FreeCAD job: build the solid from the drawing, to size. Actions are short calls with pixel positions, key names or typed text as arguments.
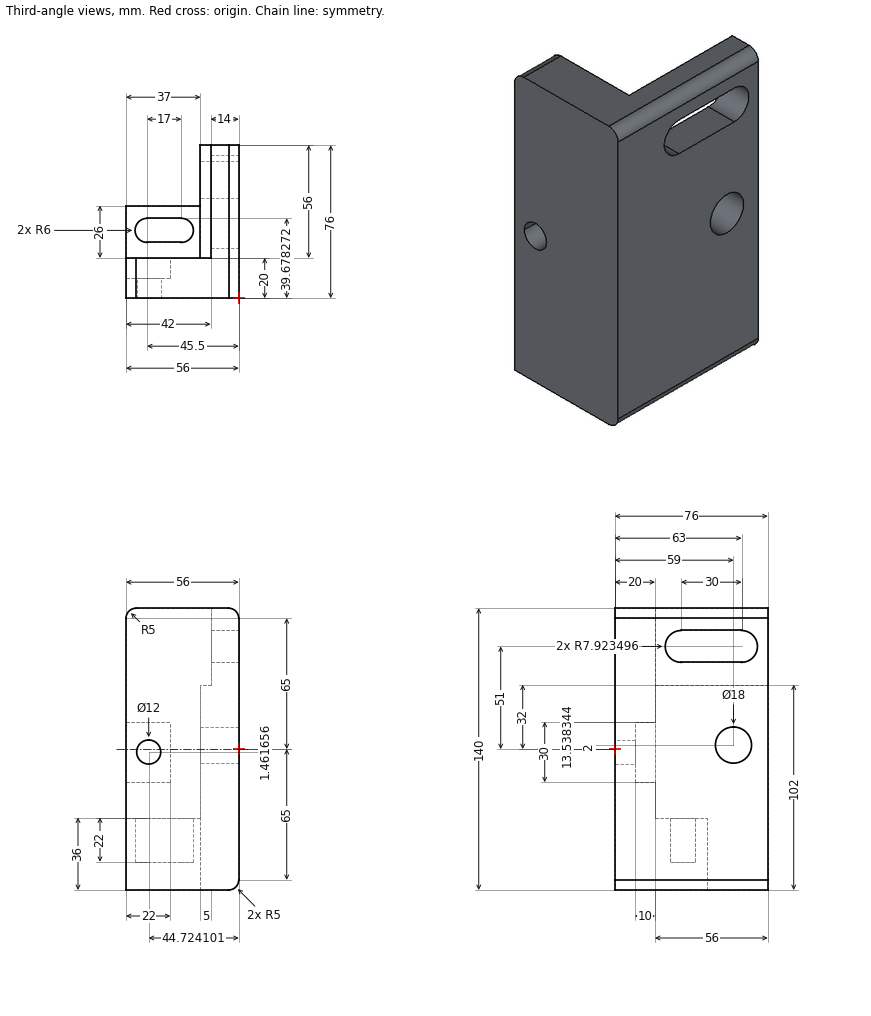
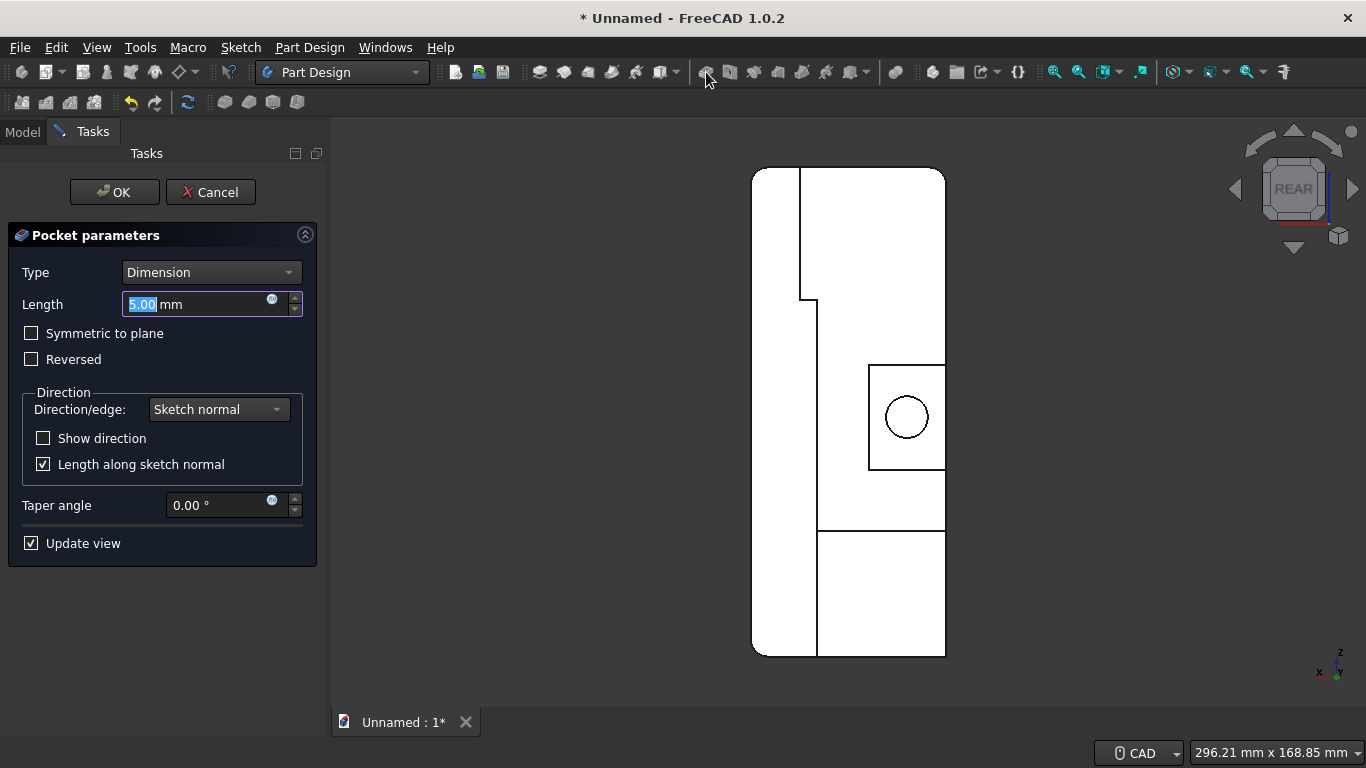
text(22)
key(Tab)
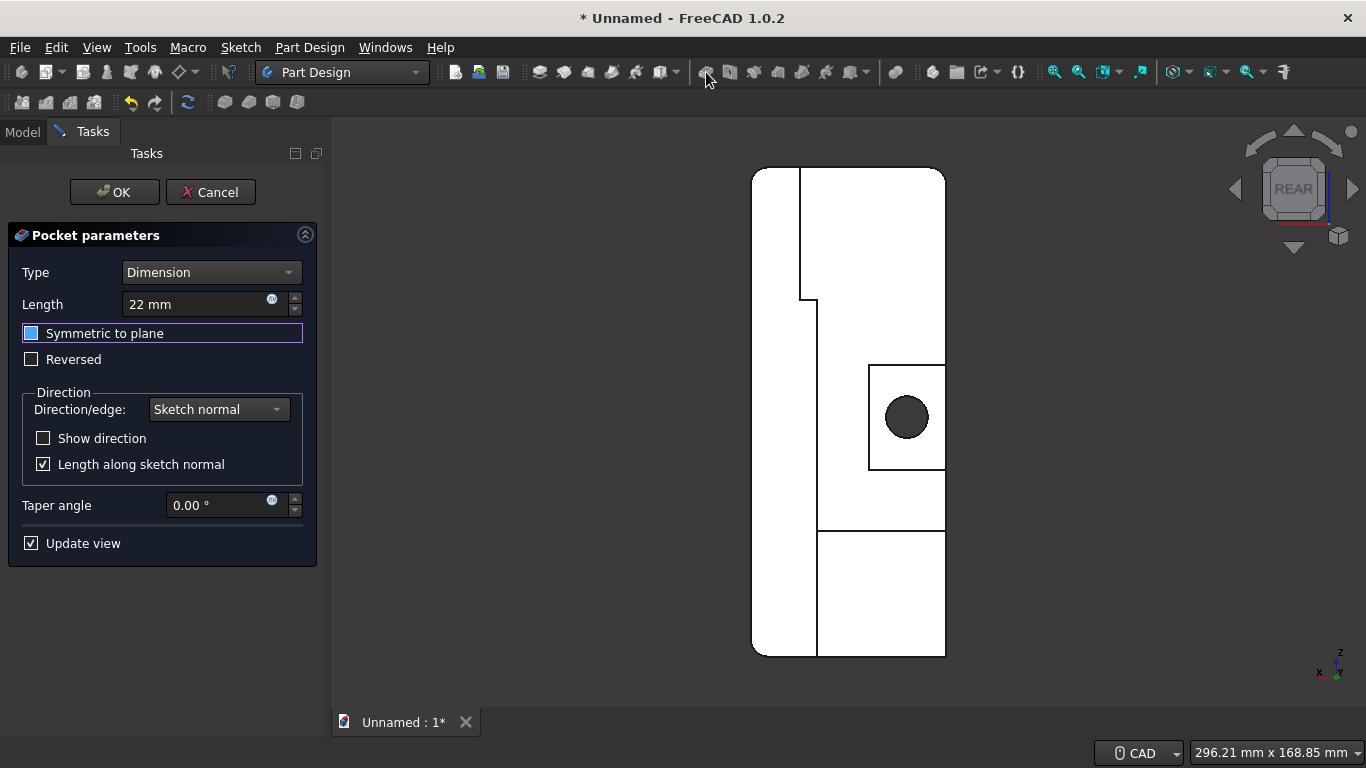
click(115, 192)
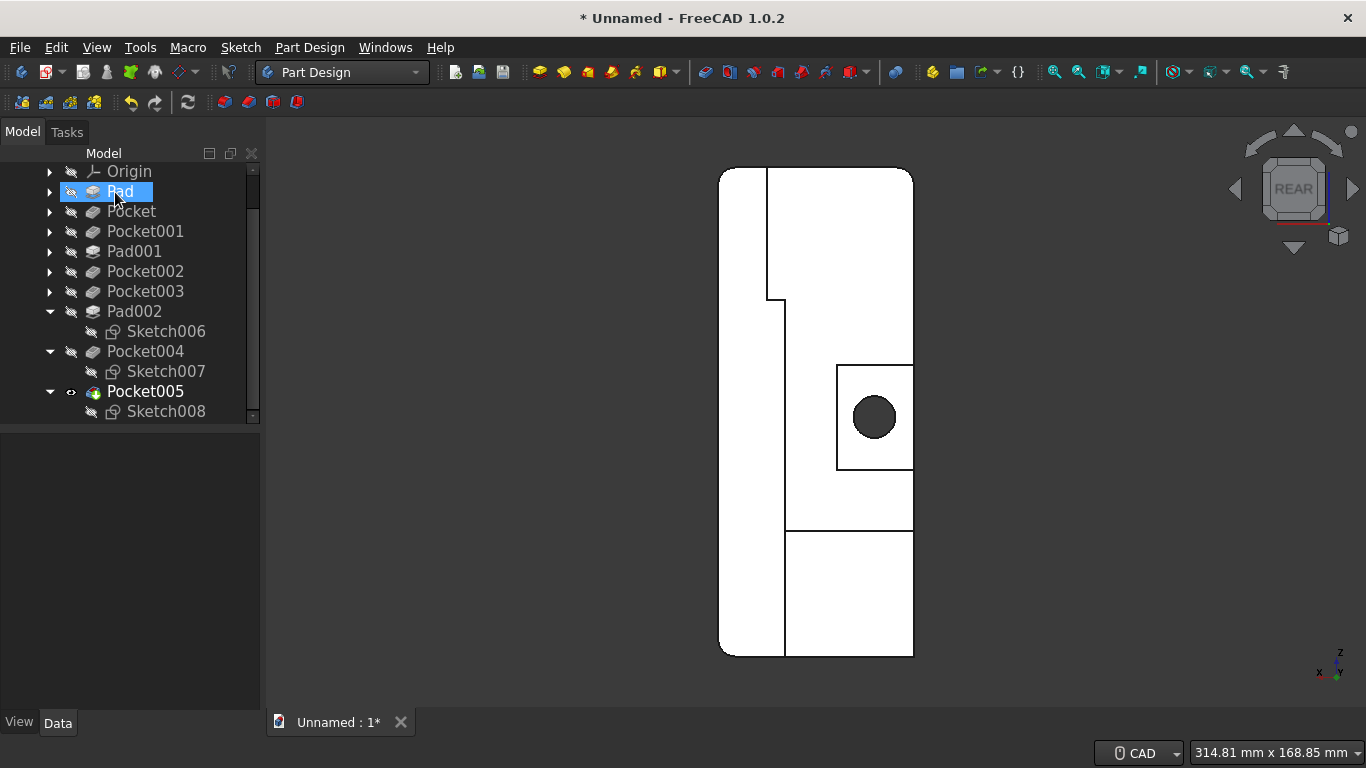
key(0)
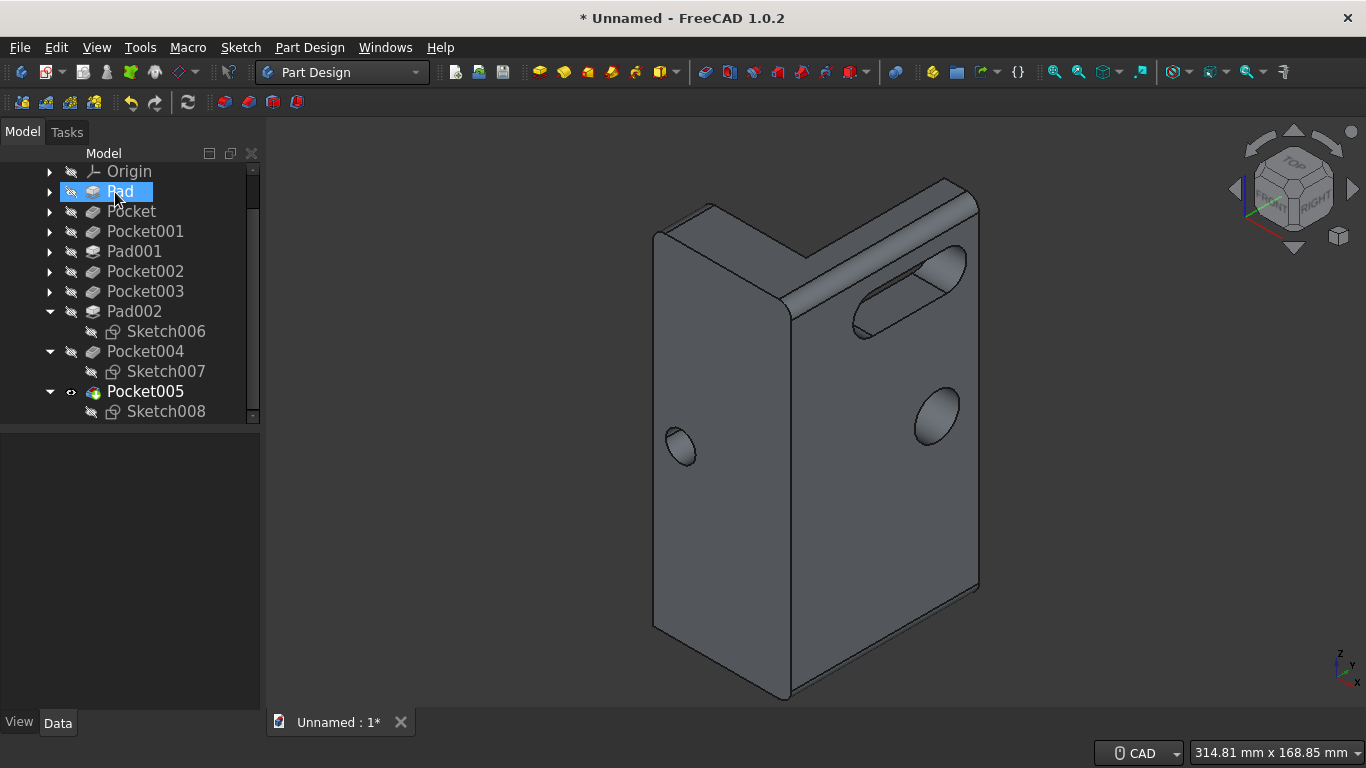
key(2)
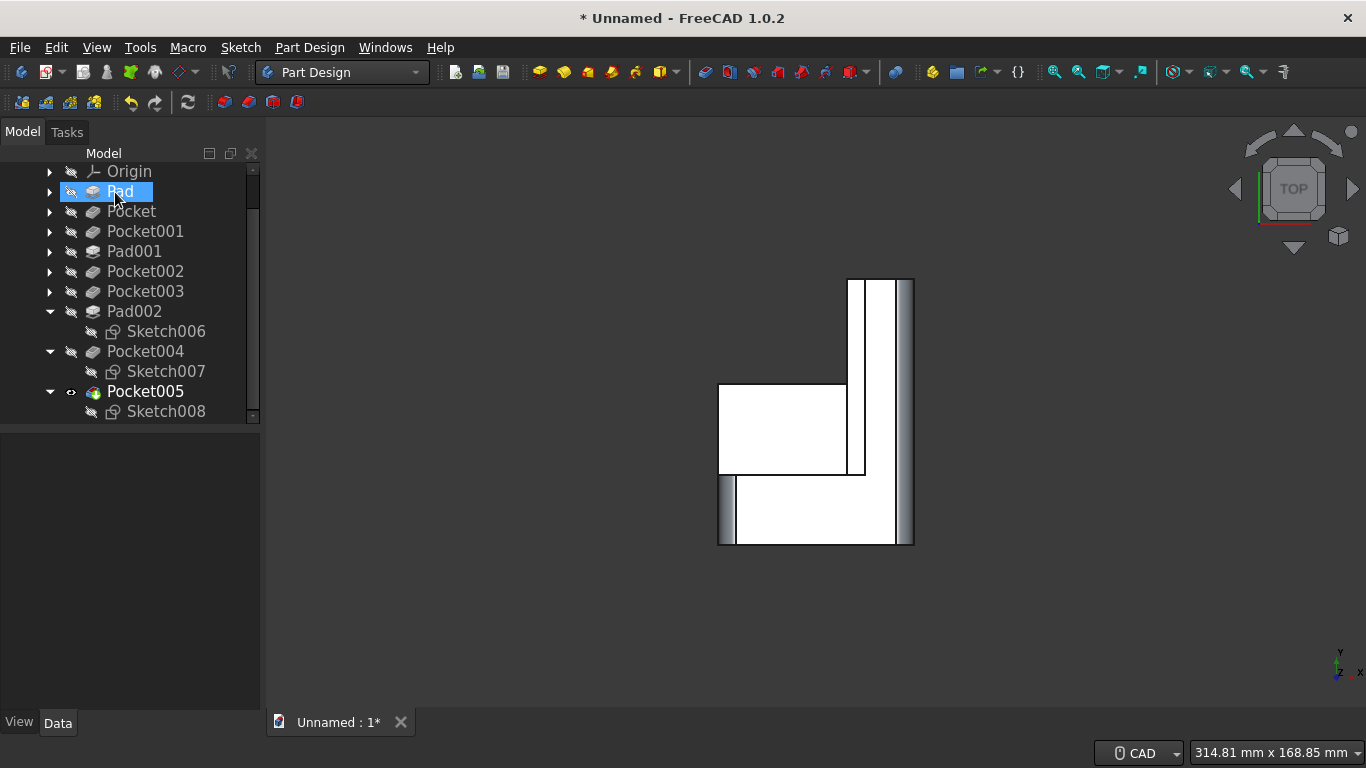
click(801, 428)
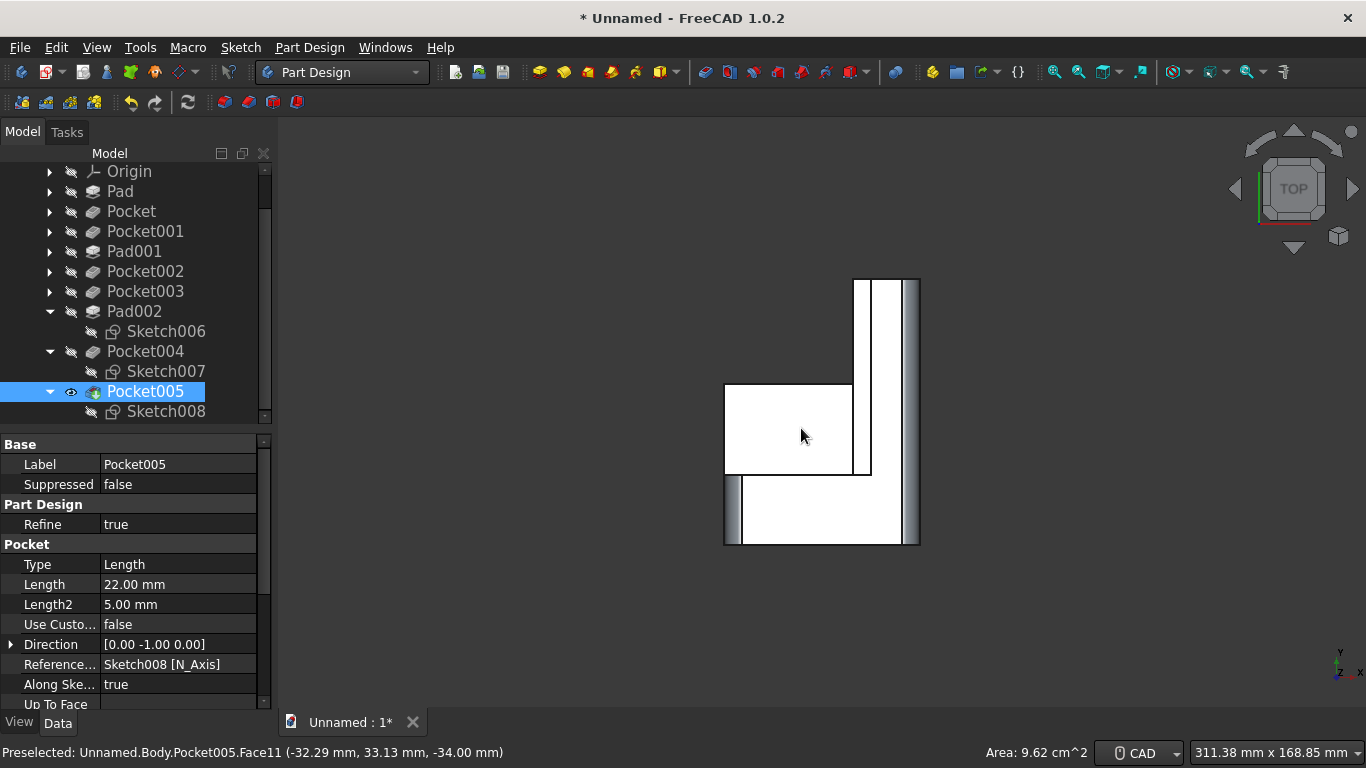
click(46, 72)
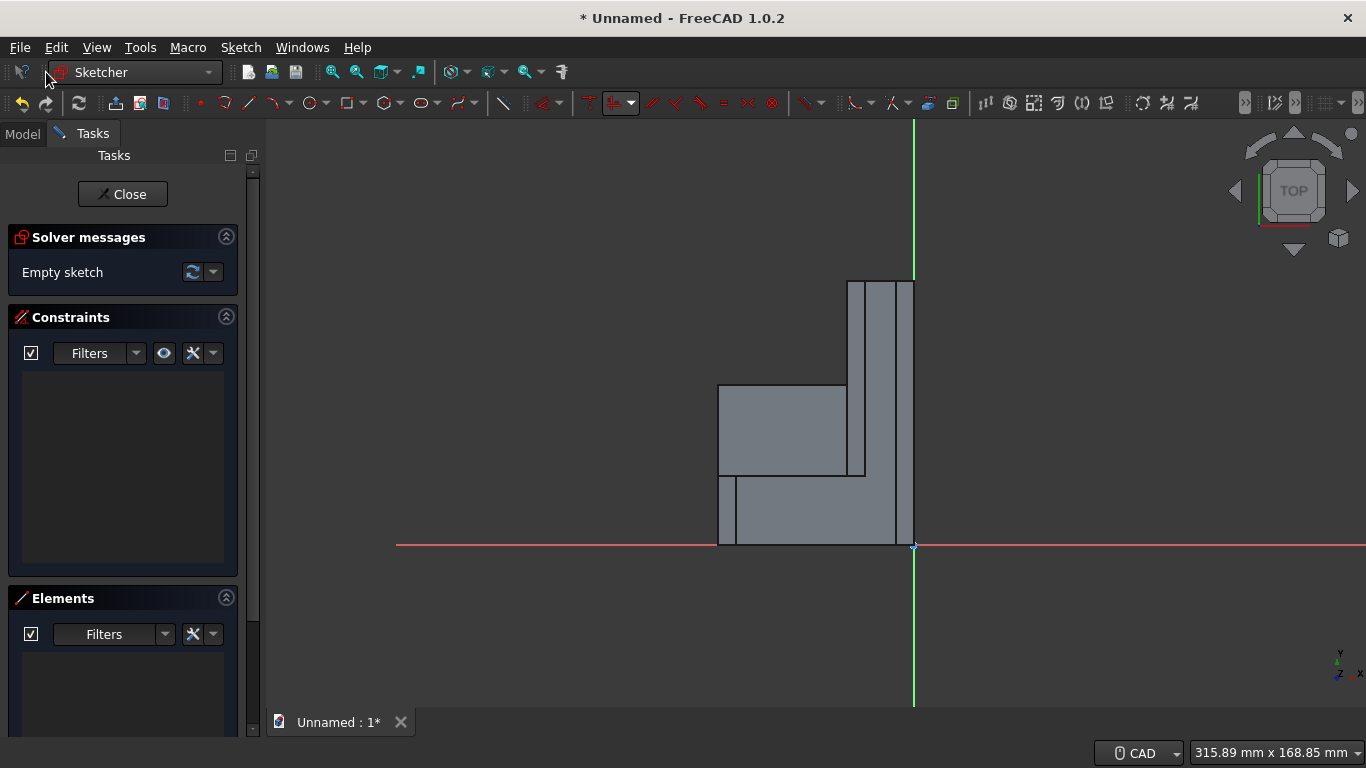
click(164, 104)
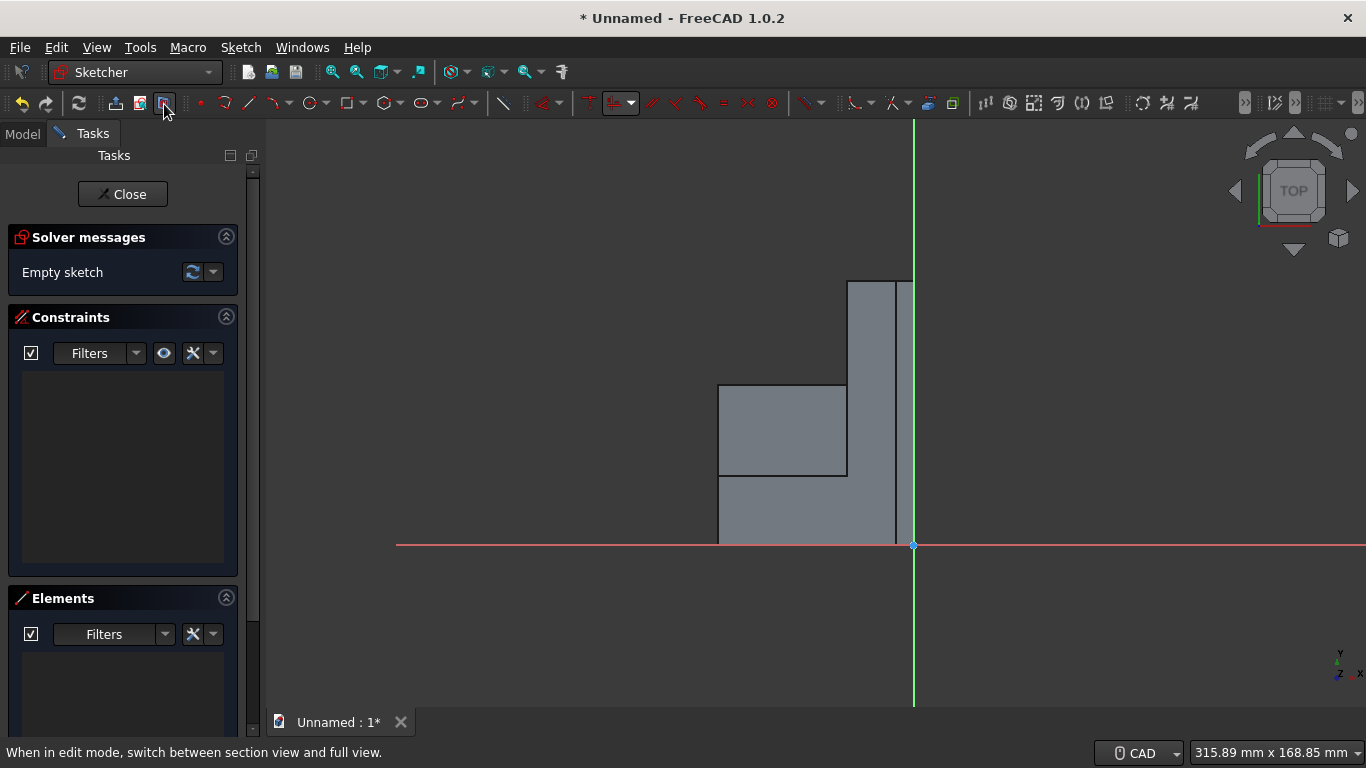
scroll(868, 513, up, 5)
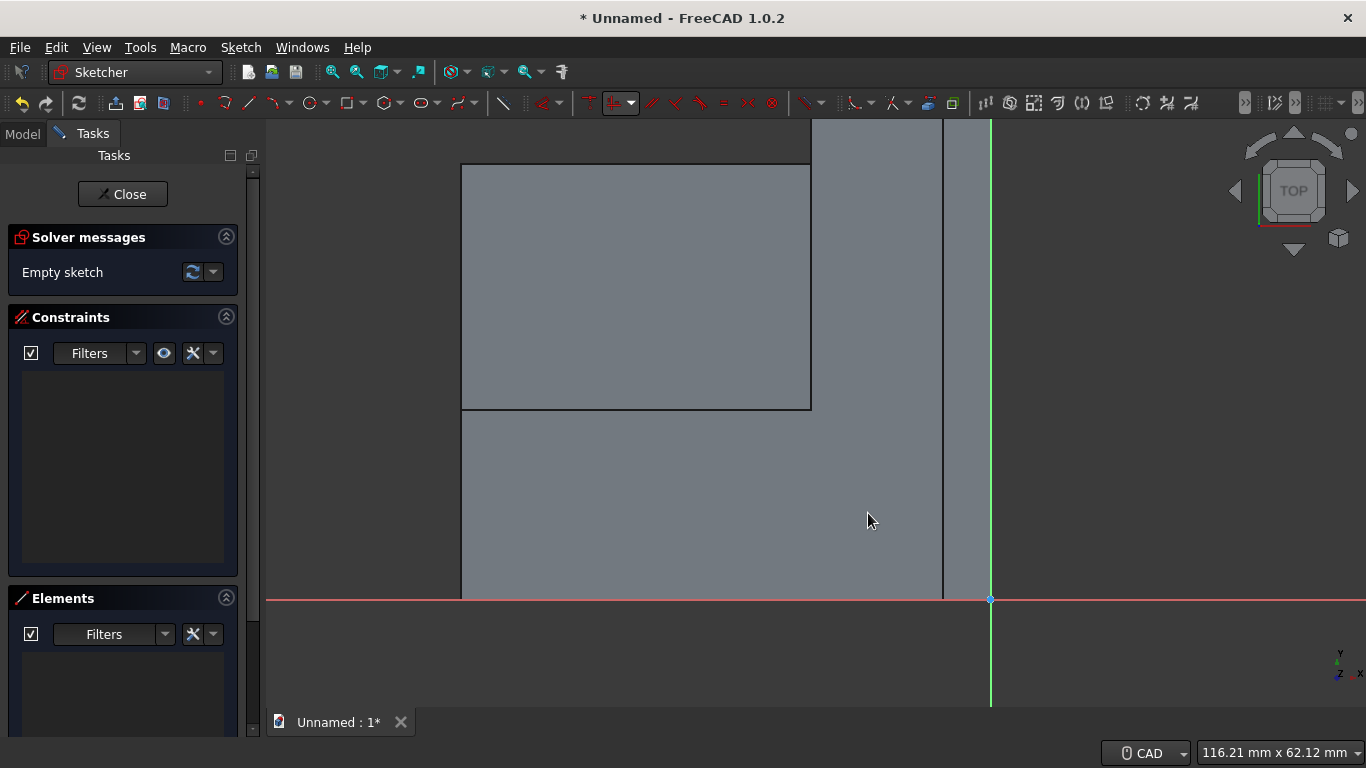
click(422, 104)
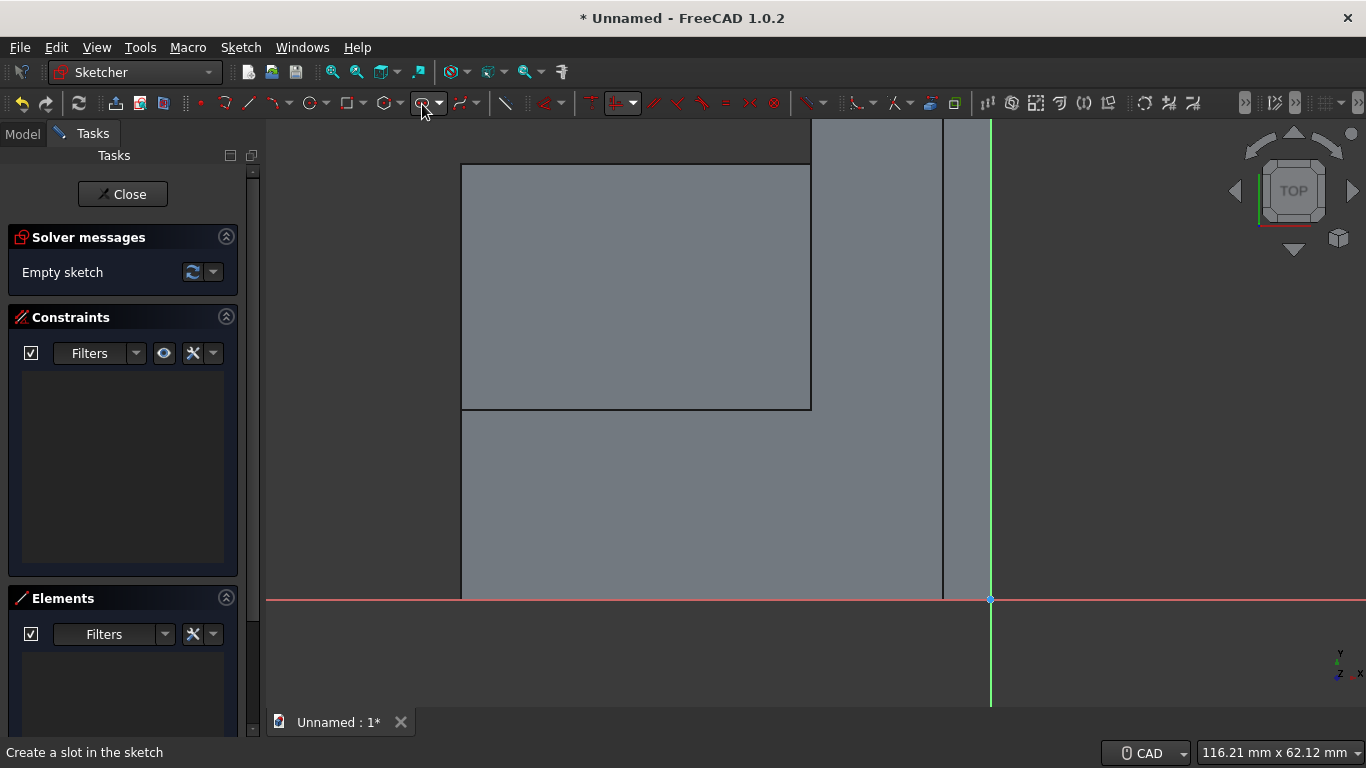
click(560, 281)